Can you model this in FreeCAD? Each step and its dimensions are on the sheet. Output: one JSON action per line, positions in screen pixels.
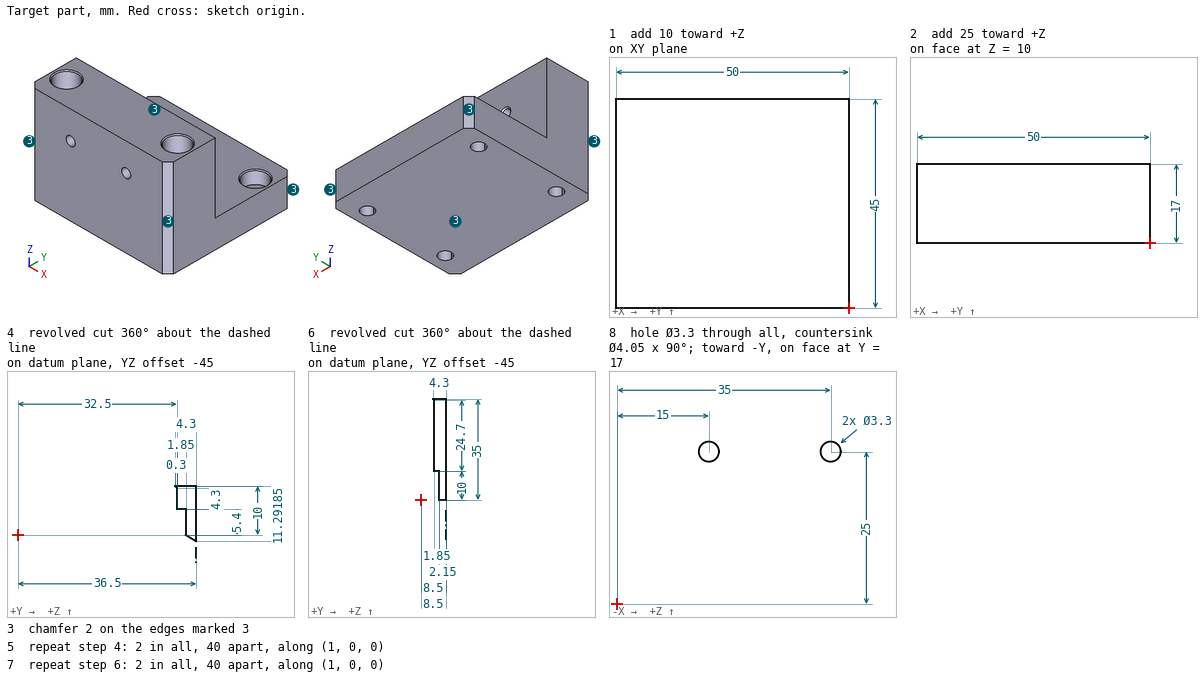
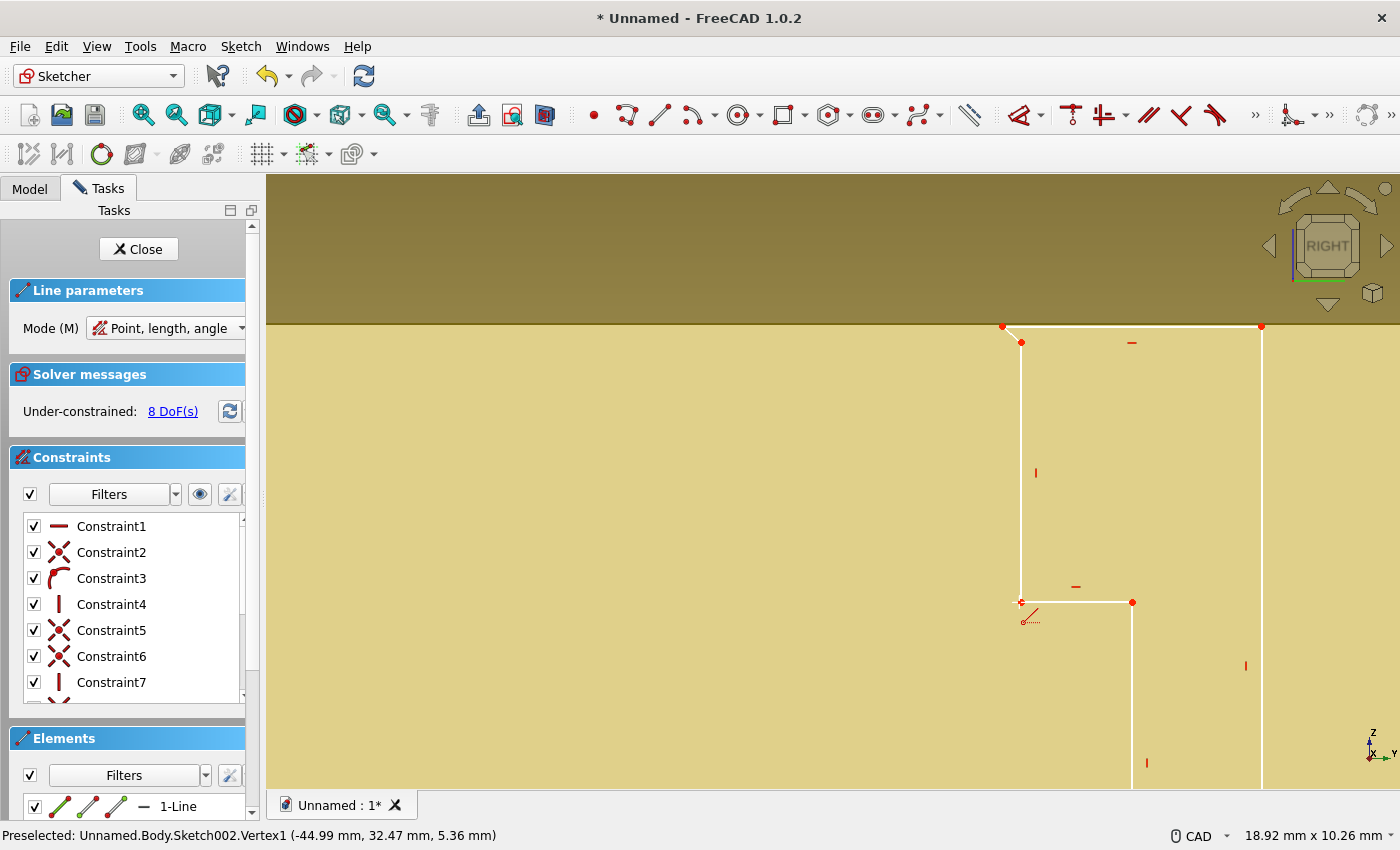
{"action": "scroll", "coordinate": [1022, 345], "scroll_direction": "down", "scroll_amount": 6}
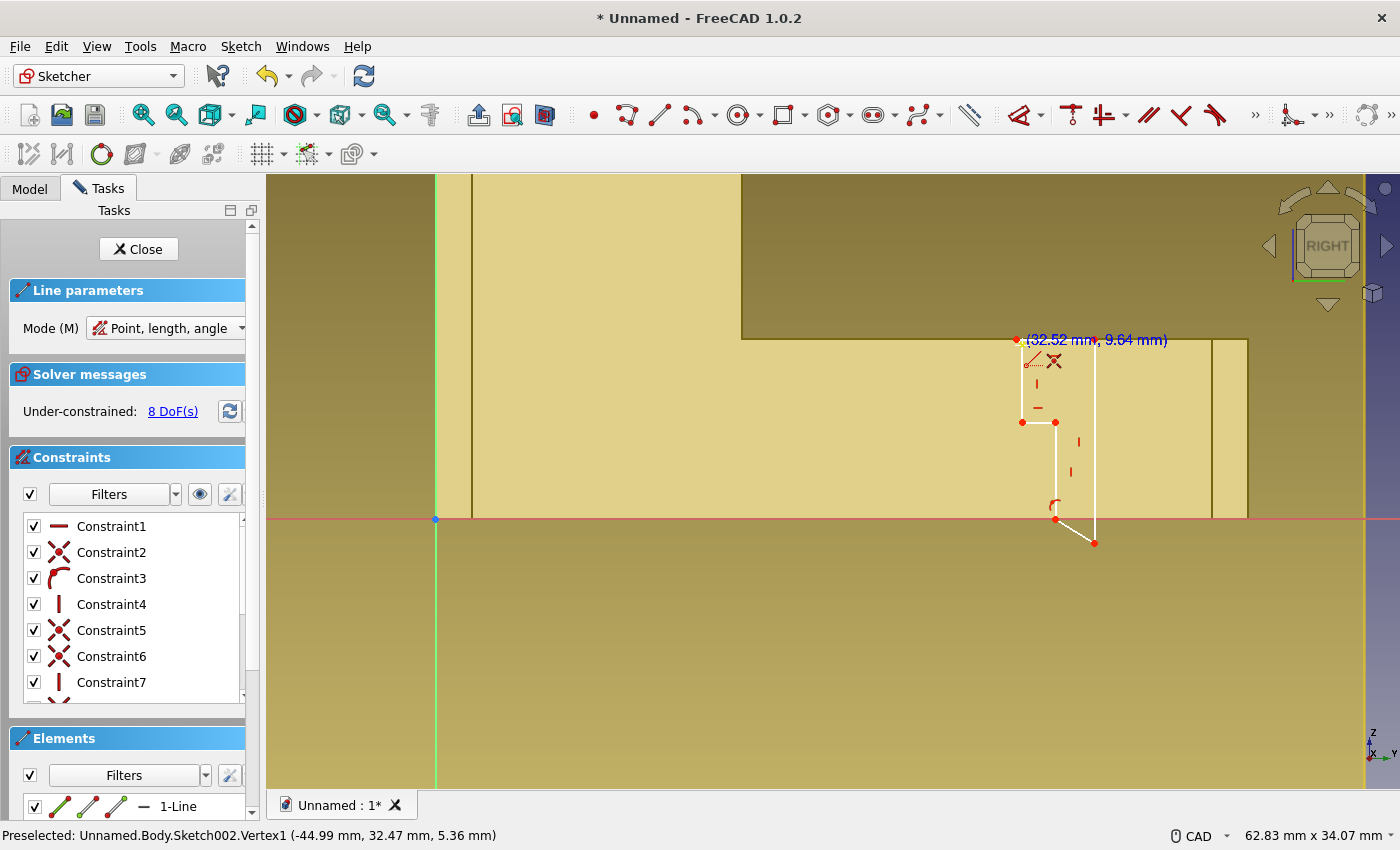
{"action": "left_click", "coordinate": [1094, 563]}
{"action": "left_click", "coordinate": [1094, 624]}
{"action": "key", "text": "Escape"}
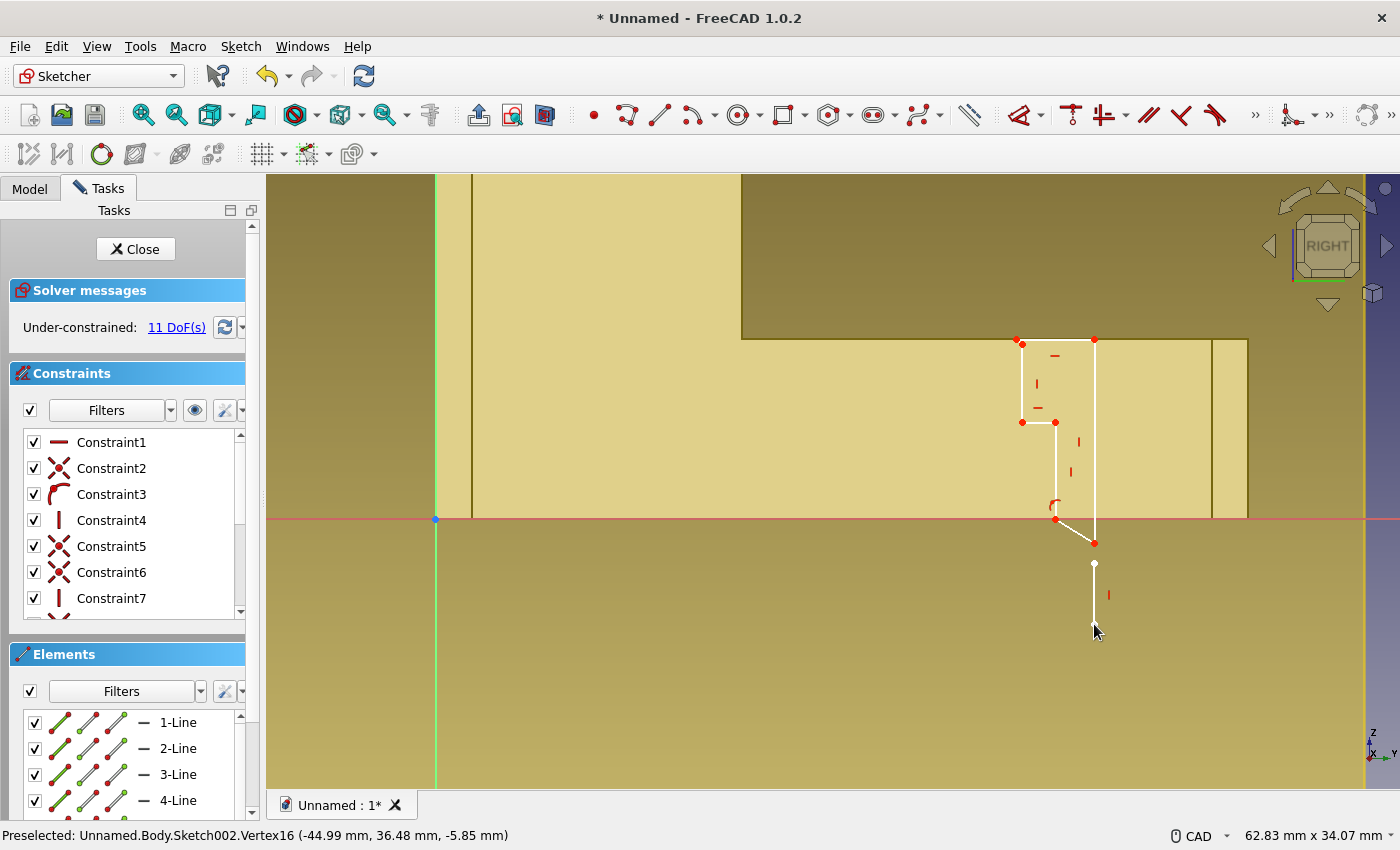
{"action": "left_click", "coordinate": [1094, 582]}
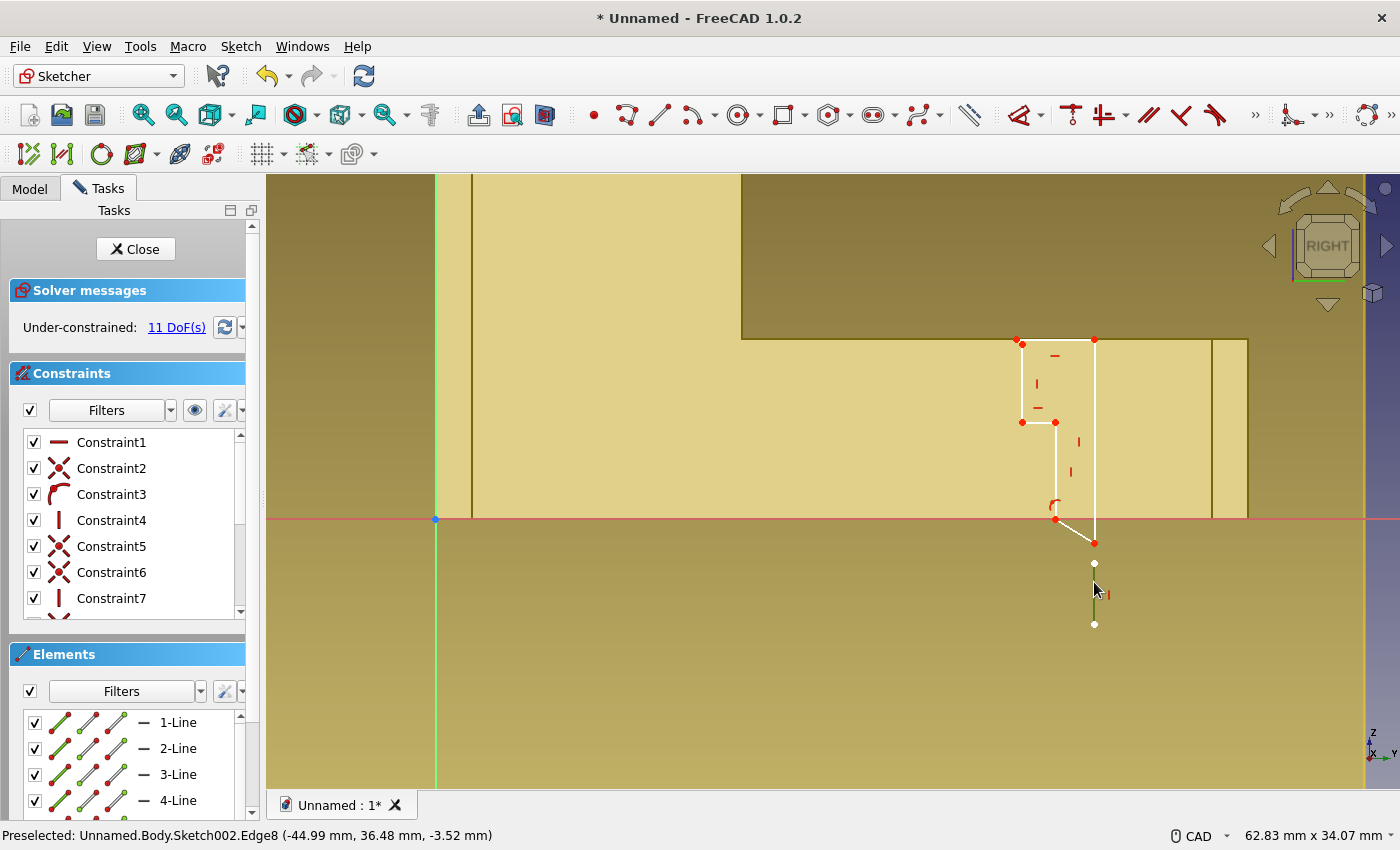
{"action": "key", "text": "g n"}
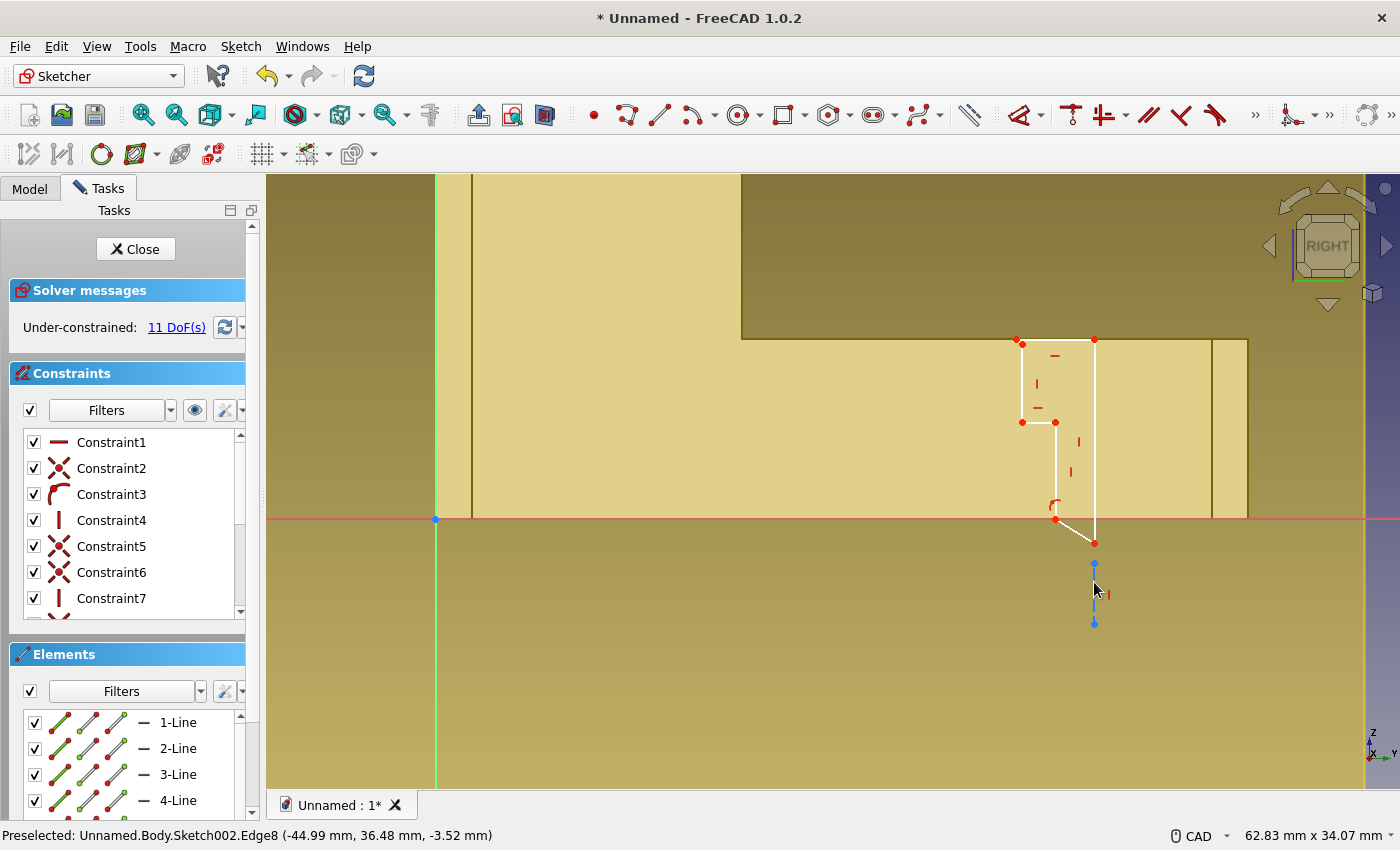
{"action": "left_click", "coordinate": [1056, 452]}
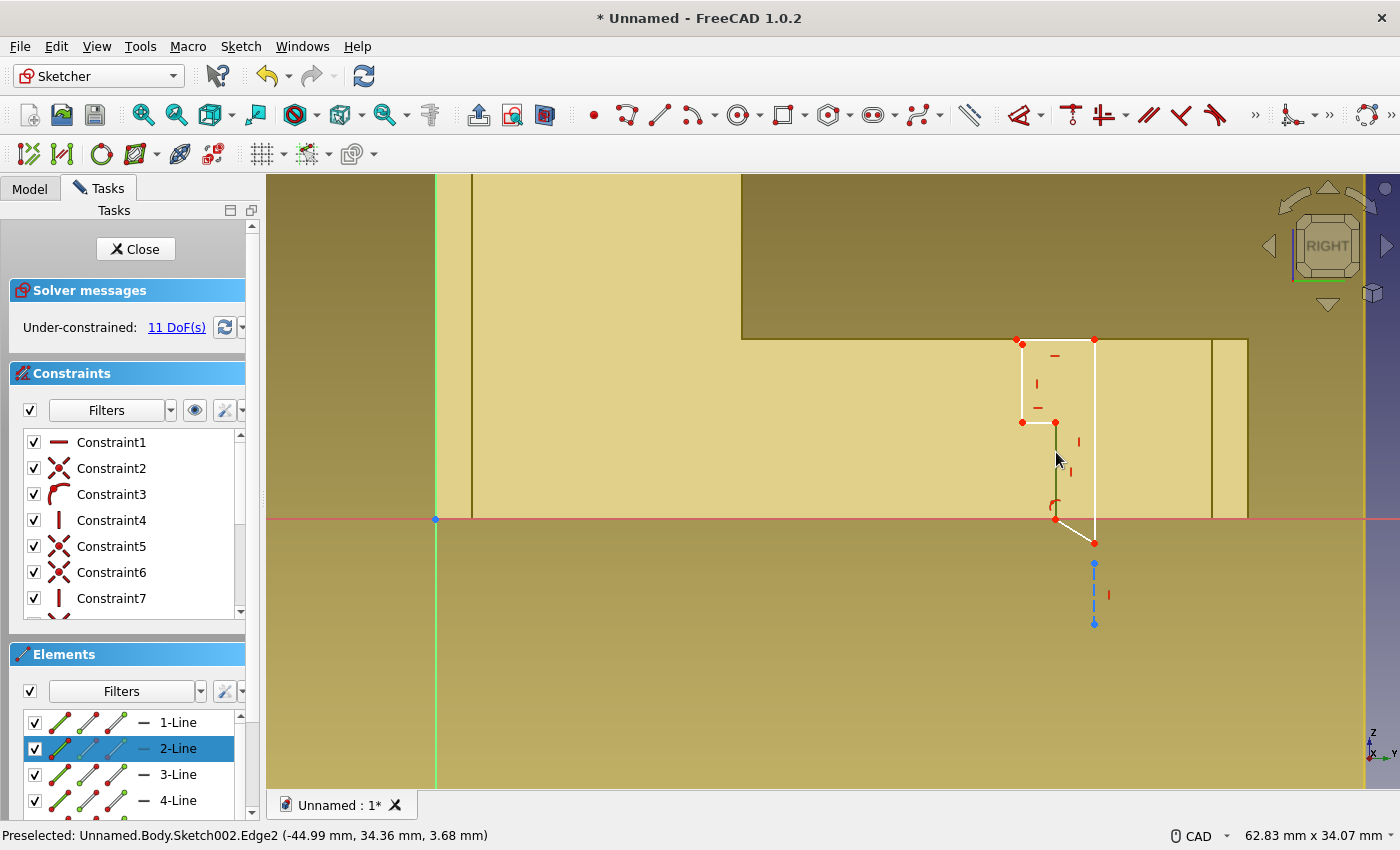
{"action": "key", "text": "i"}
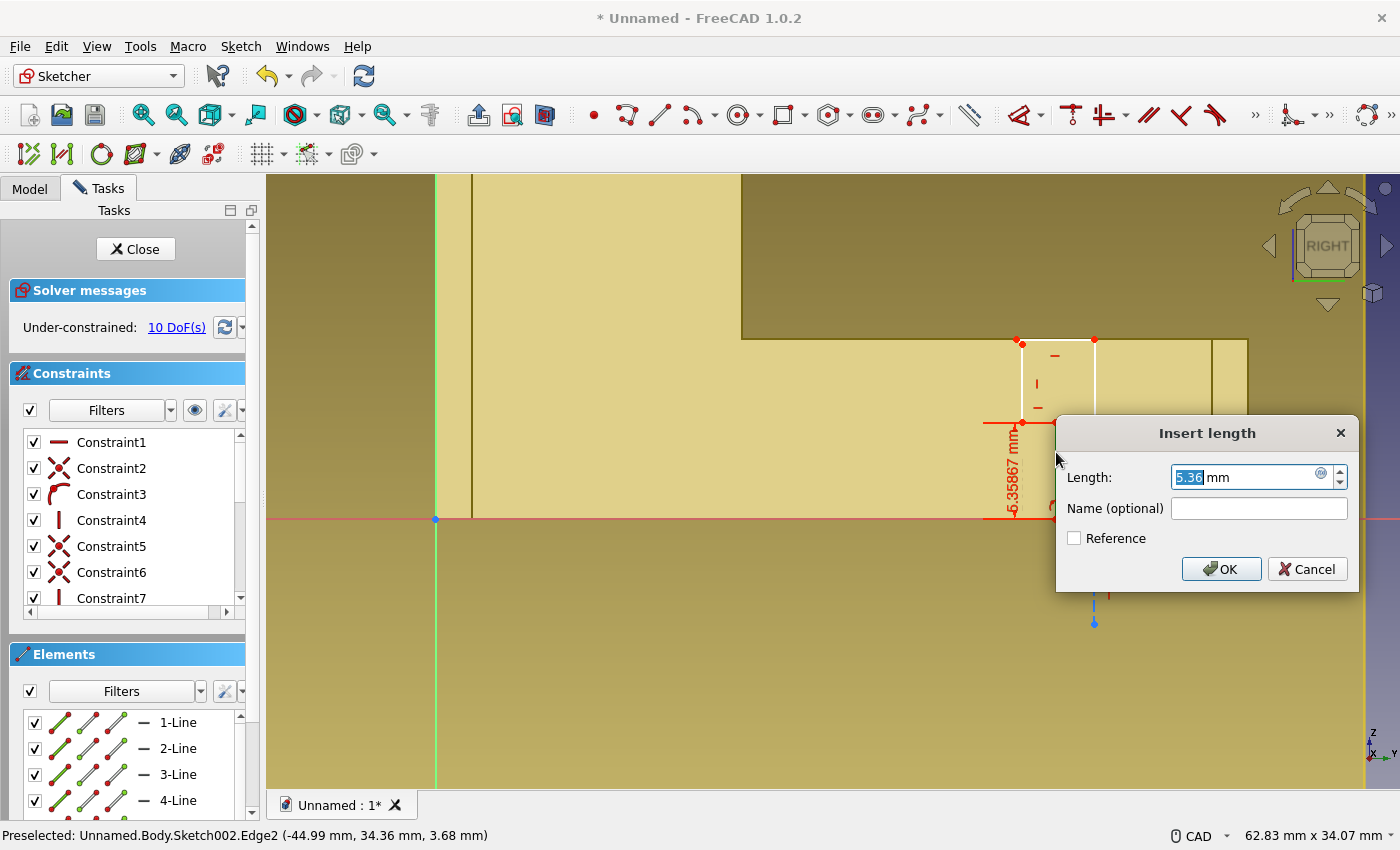
{"action": "type", "text": "5.4"}
{"action": "key", "text": "Return"}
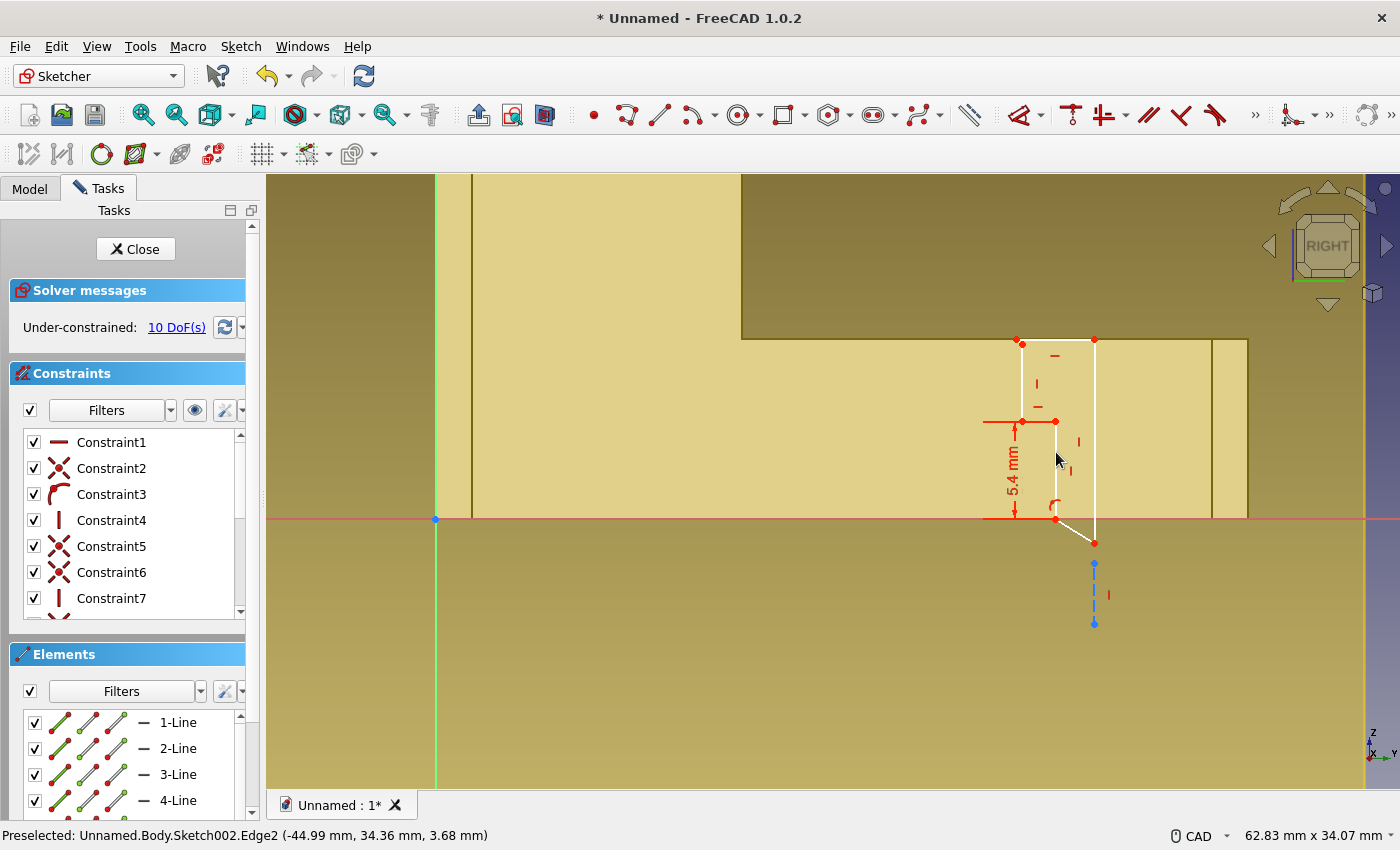
{"action": "left_click", "coordinate": [1071, 340]}